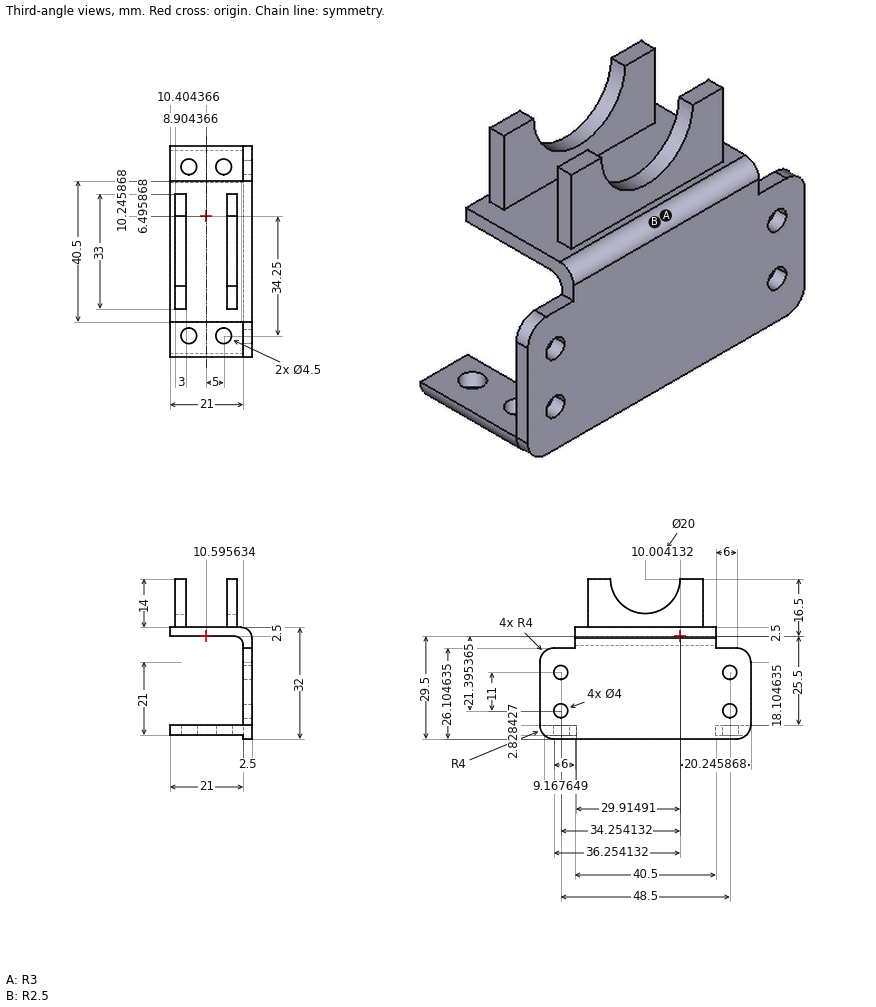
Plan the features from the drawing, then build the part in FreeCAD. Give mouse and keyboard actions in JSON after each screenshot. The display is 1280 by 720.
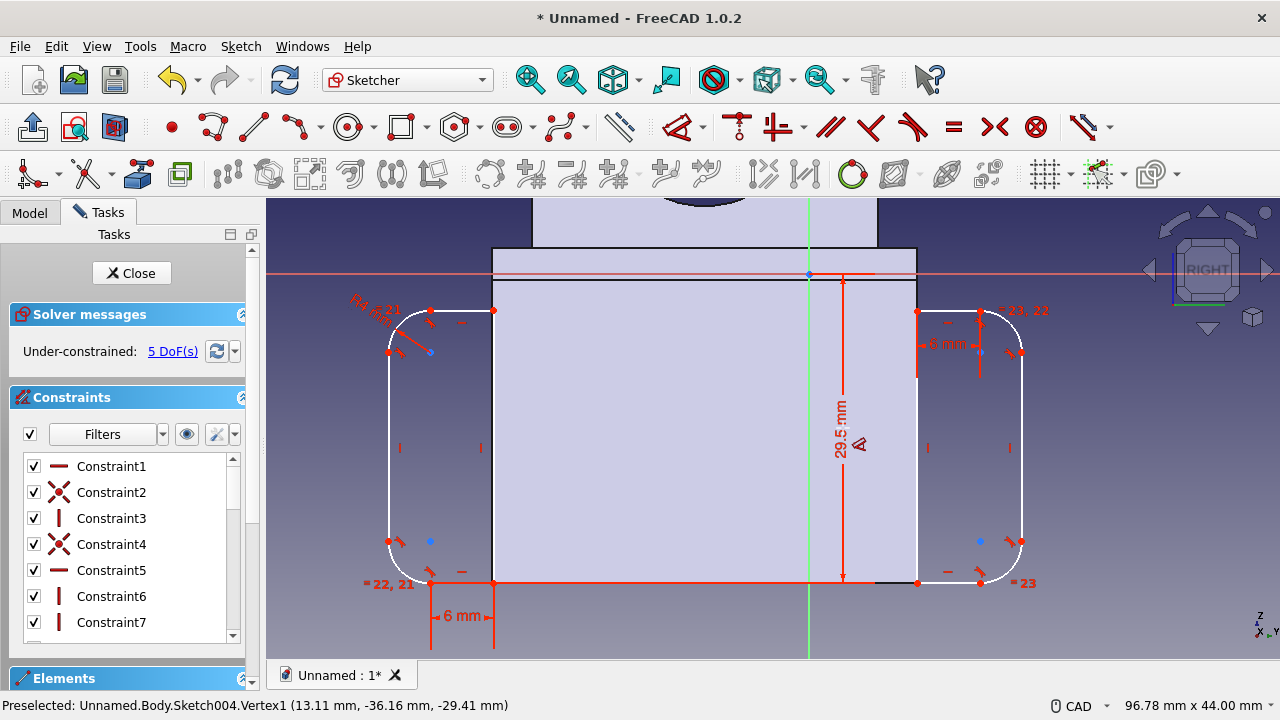
{"action": "left_click", "coordinate": [1022, 541]}
{"action": "left_click", "coordinate": [1056, 408]}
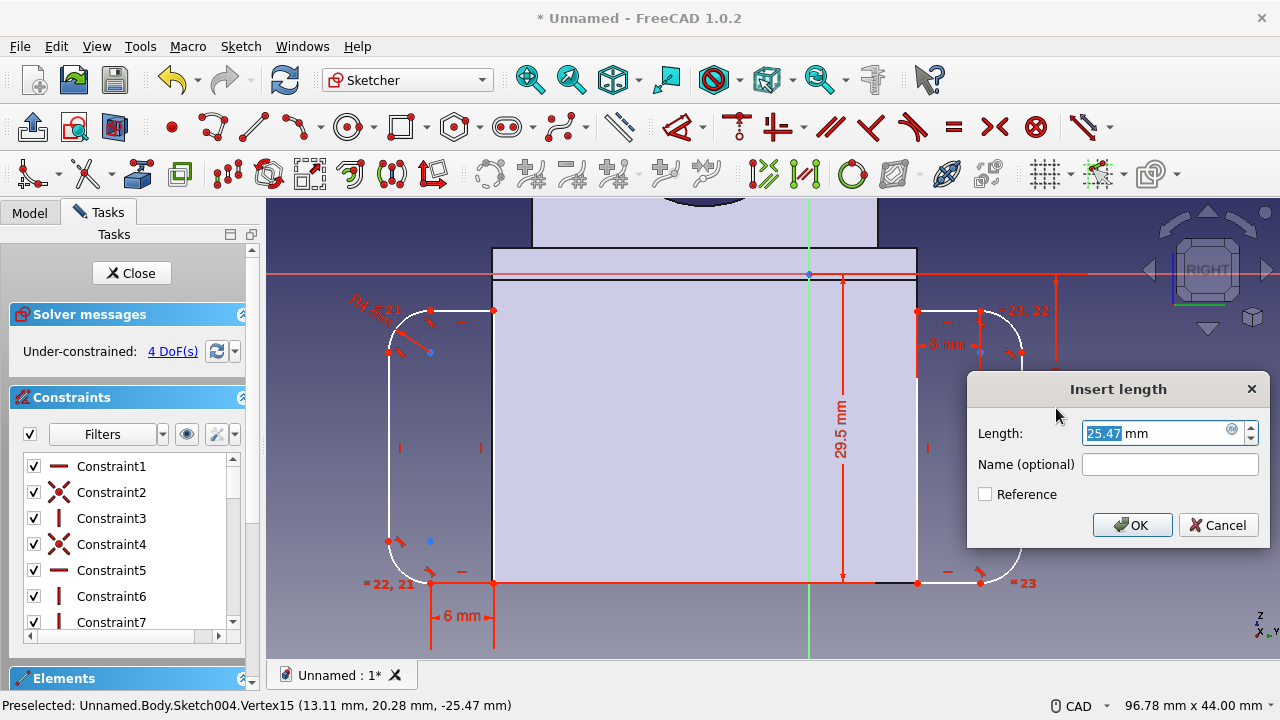
{"action": "type", "text": "25.5"}
{"action": "key", "text": "Return"}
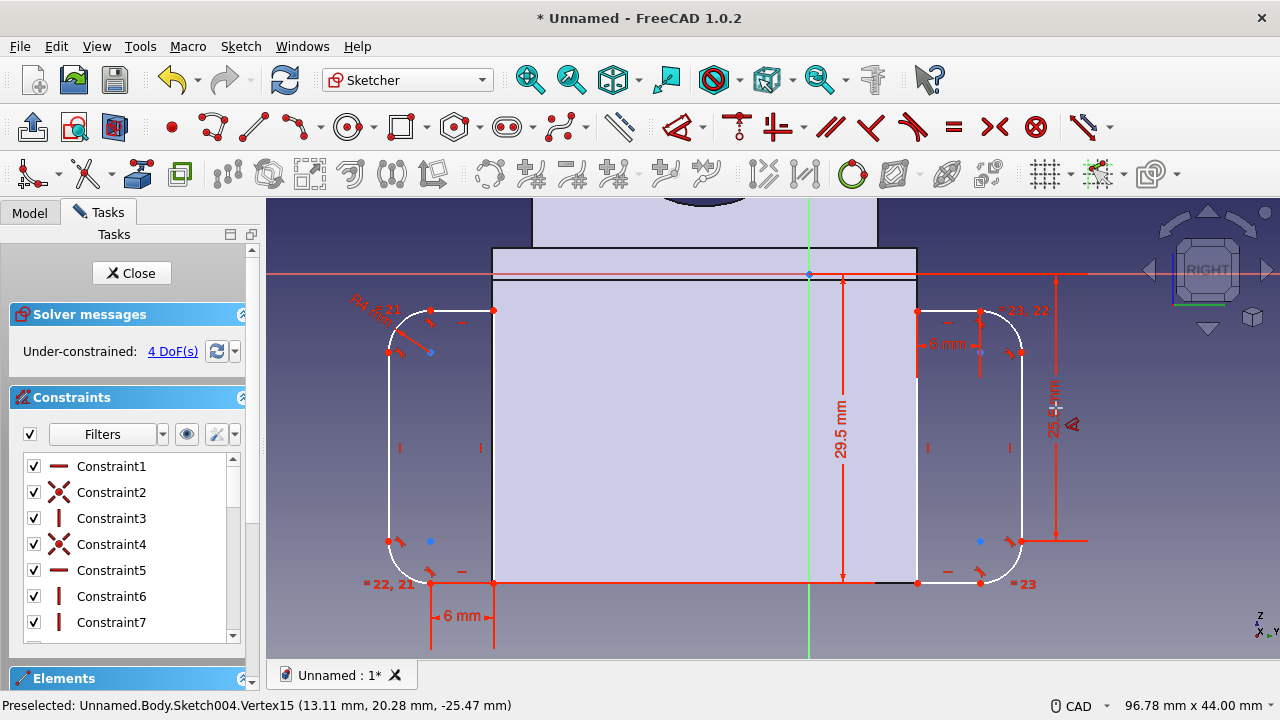
{"action": "left_click", "coordinate": [494, 502]}
{"action": "left_click", "coordinate": [460, 447]}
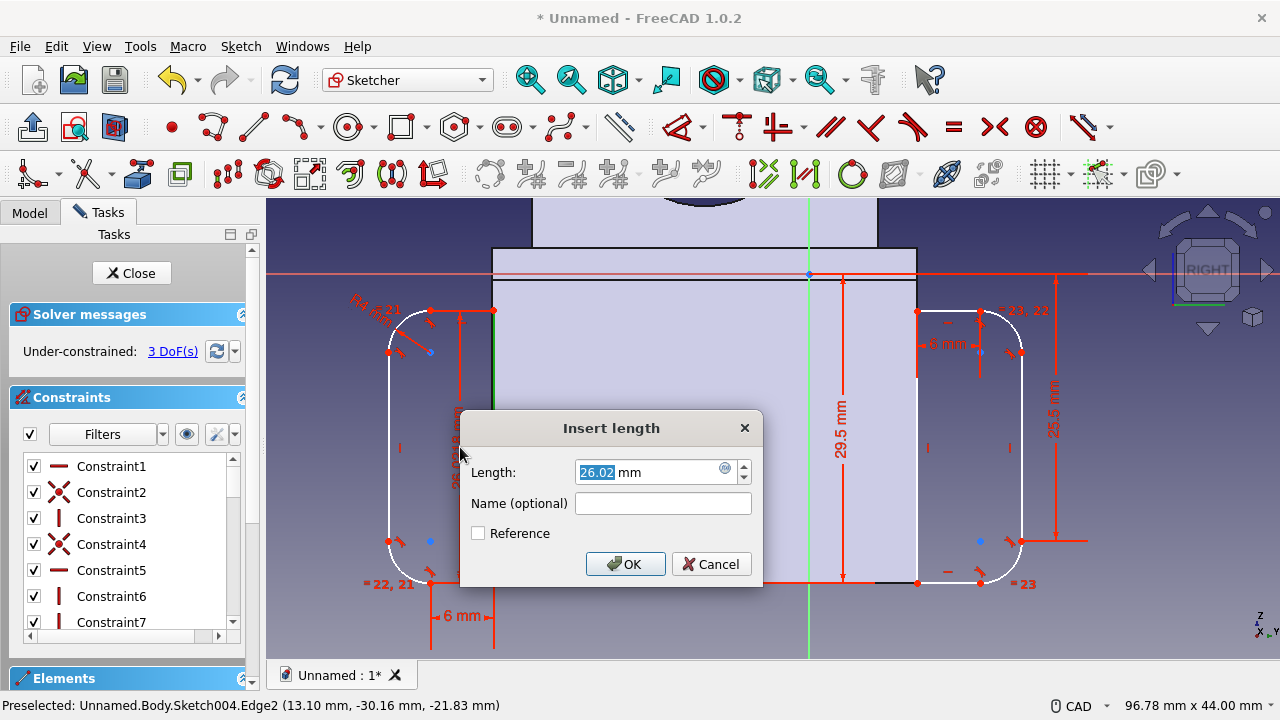
{"action": "type", "text": "26.104635"}
{"action": "key", "text": "Return"}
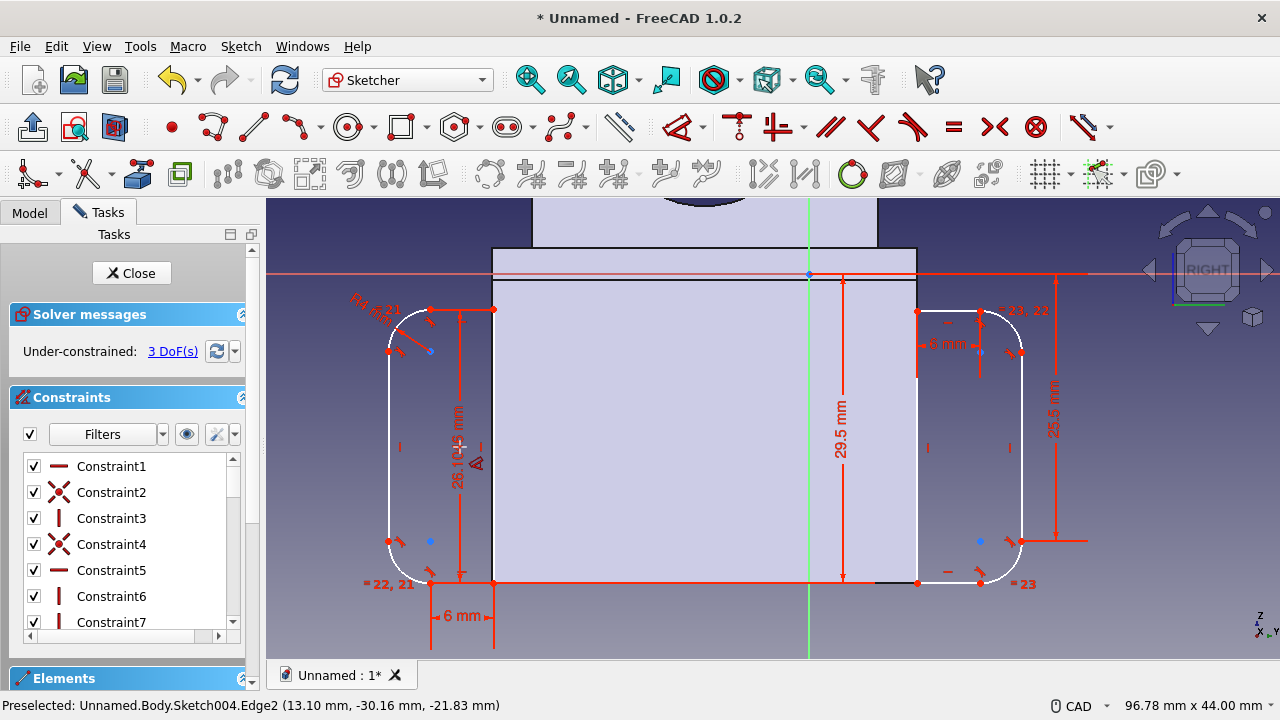
{"action": "left_click", "coordinate": [1022, 485]}
{"action": "left_click", "coordinate": [1056, 447]}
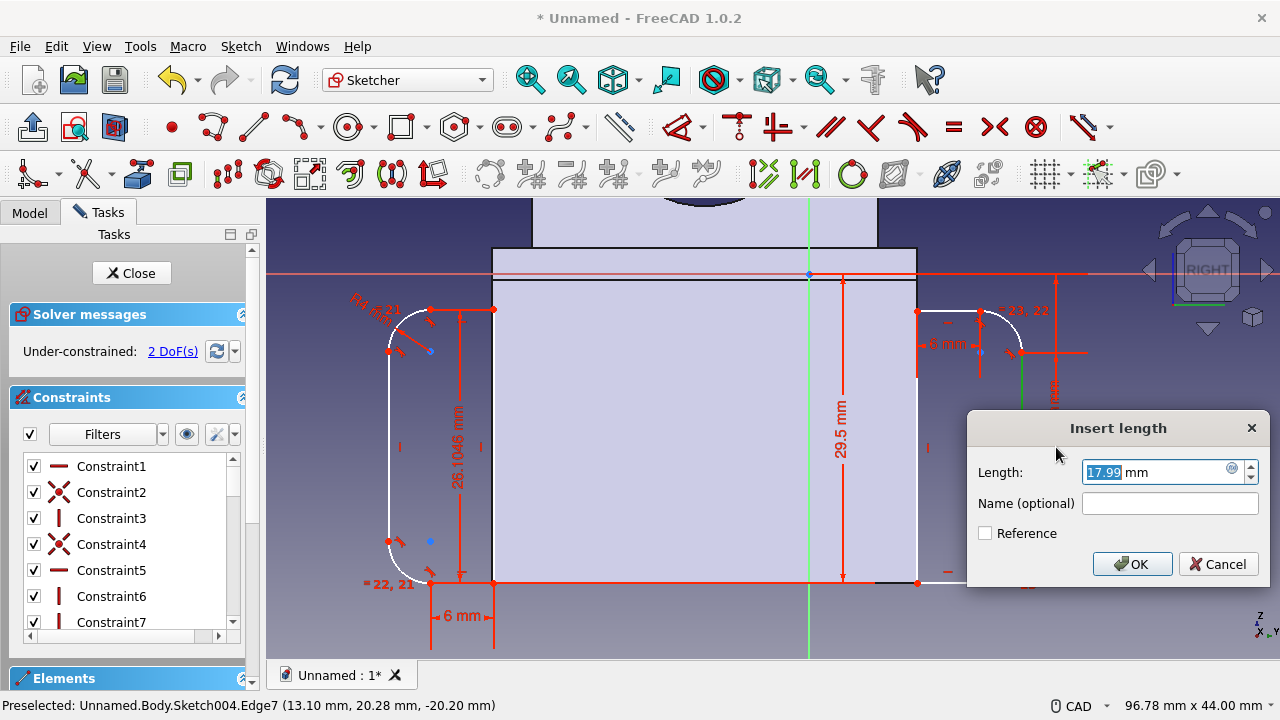
{"action": "type", "text": "18.104635"}
{"action": "key", "text": "Return"}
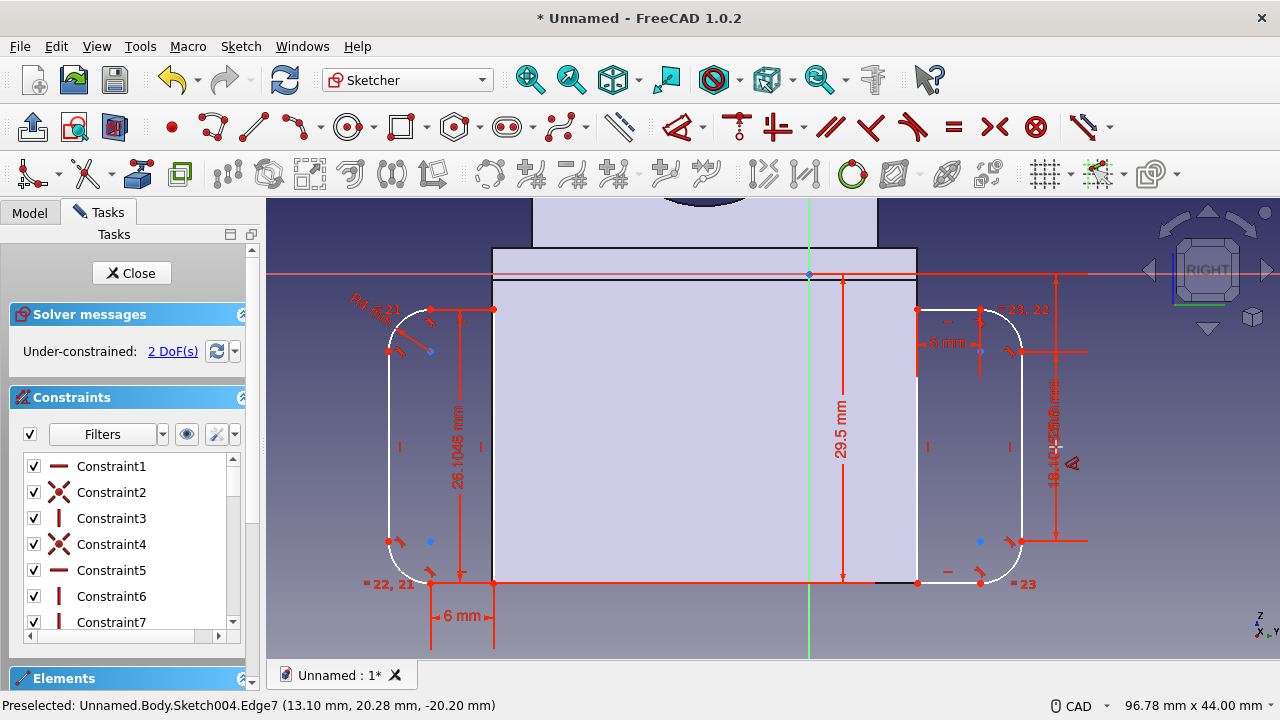
{"action": "left_click", "coordinate": [431, 583]}
{"action": "left_click", "coordinate": [620, 240]}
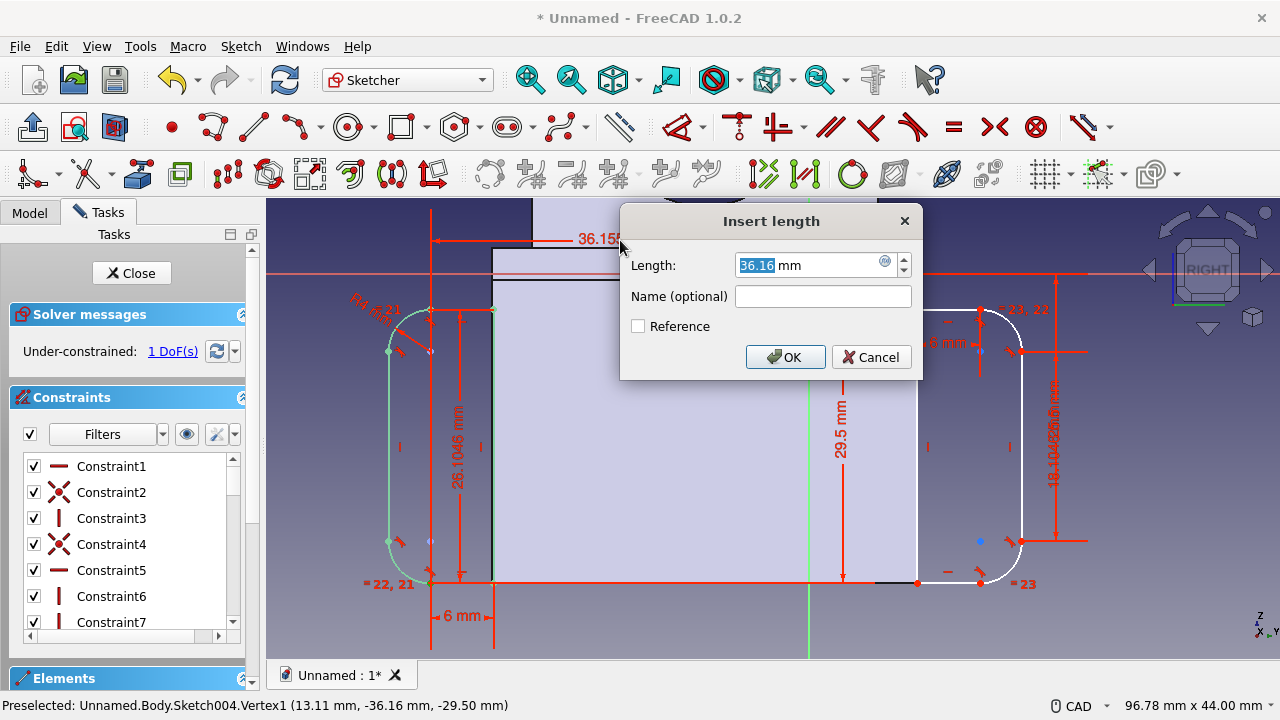
{"action": "type", "text": "36.254132"}
{"action": "key", "text": "Return"}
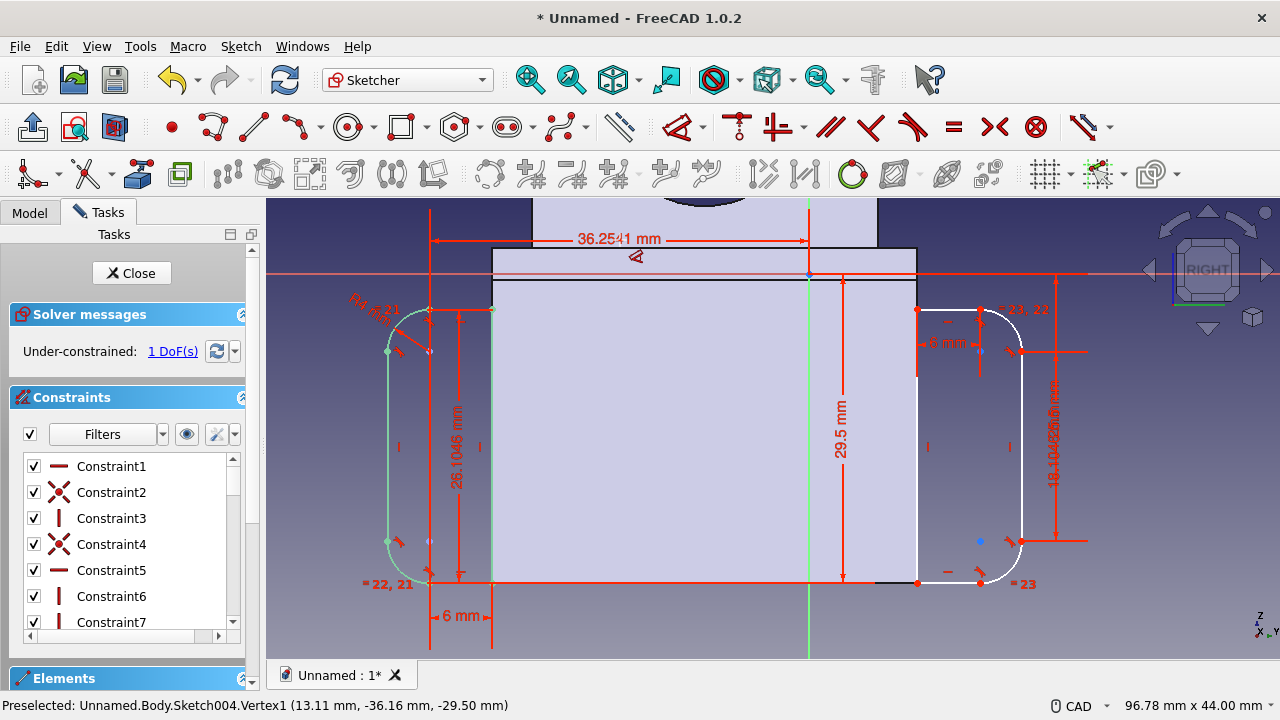
{"action": "left_click", "coordinate": [1022, 541]}
{"action": "left_click", "coordinate": [916, 240]}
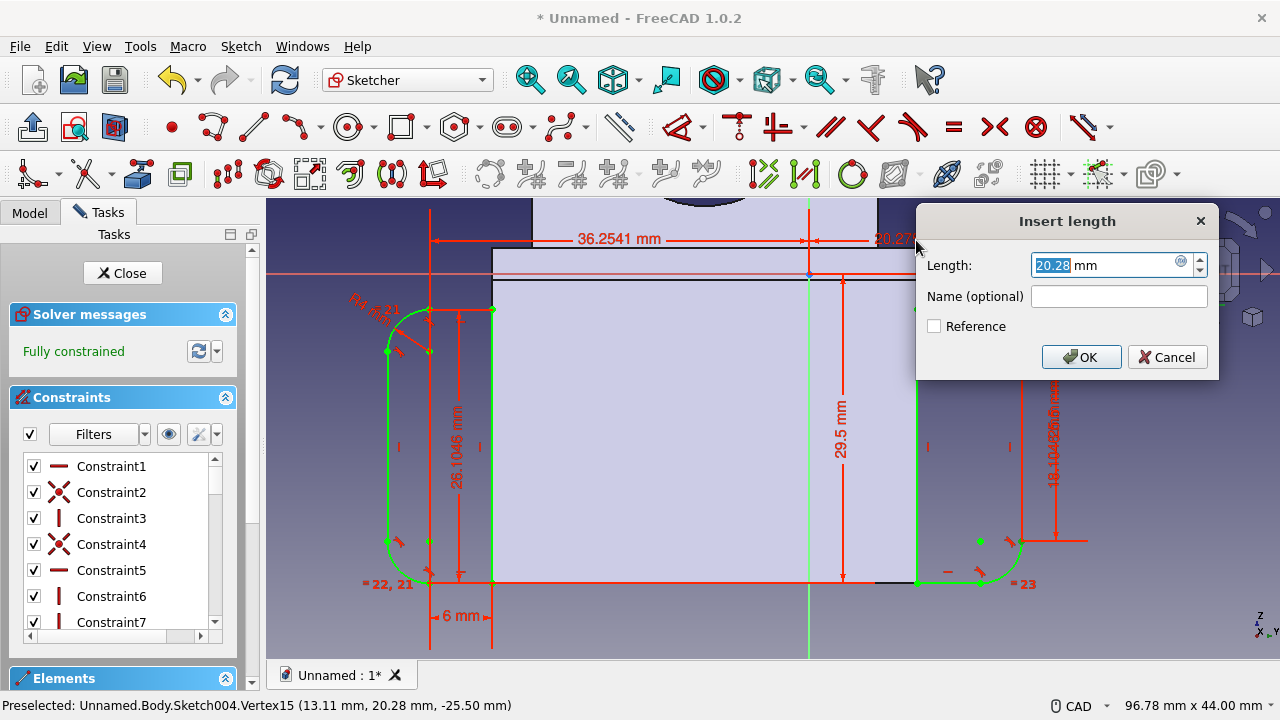
{"action": "type", "text": "20.245868"}
{"action": "key", "text": "Return"}
{"action": "key", "text": "Escape"}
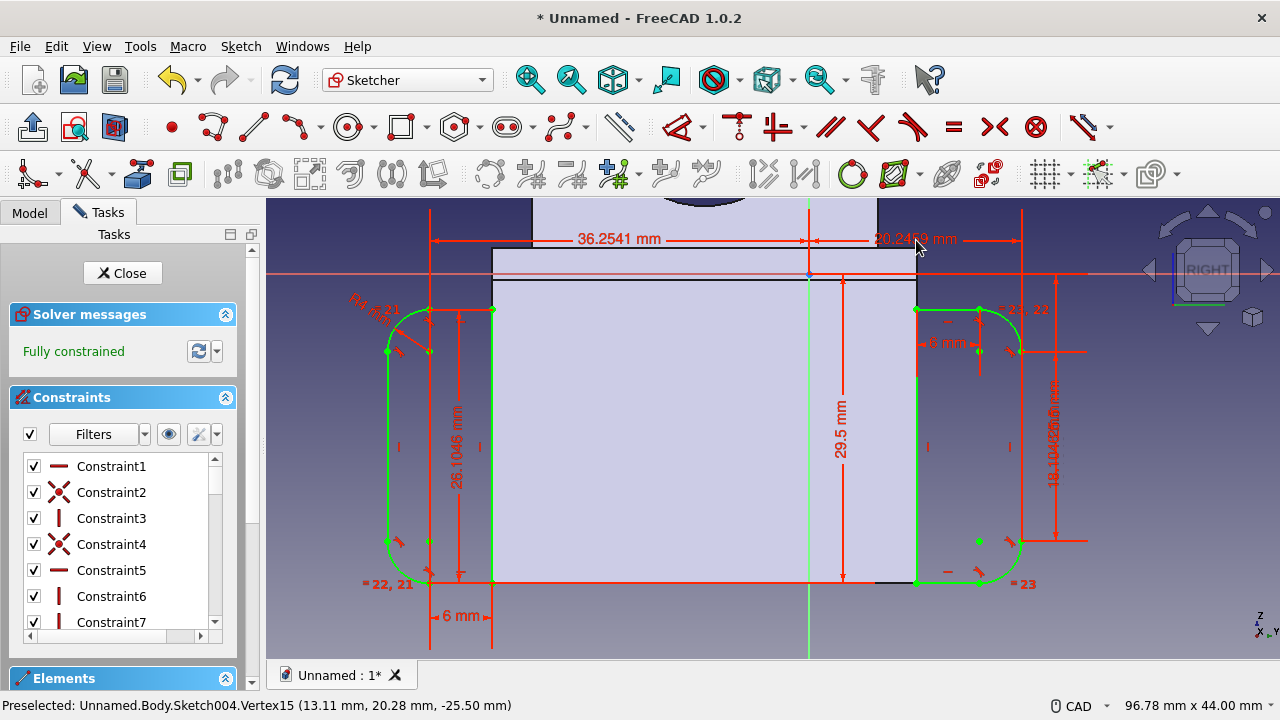
{"action": "left_click", "coordinate": [123, 273]}